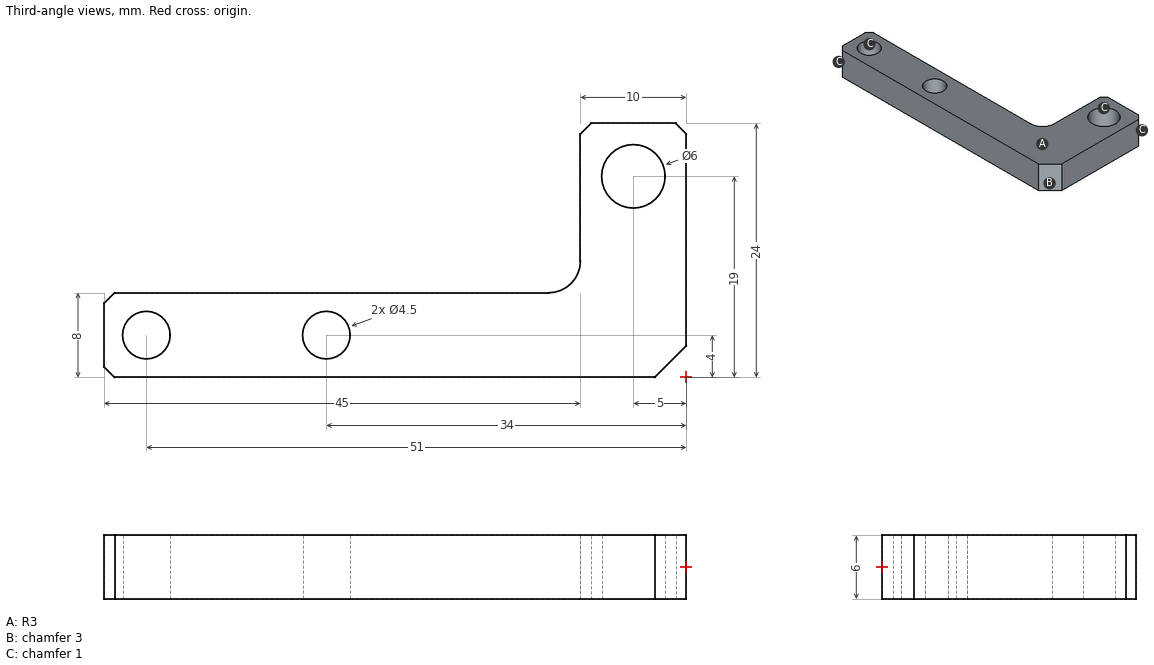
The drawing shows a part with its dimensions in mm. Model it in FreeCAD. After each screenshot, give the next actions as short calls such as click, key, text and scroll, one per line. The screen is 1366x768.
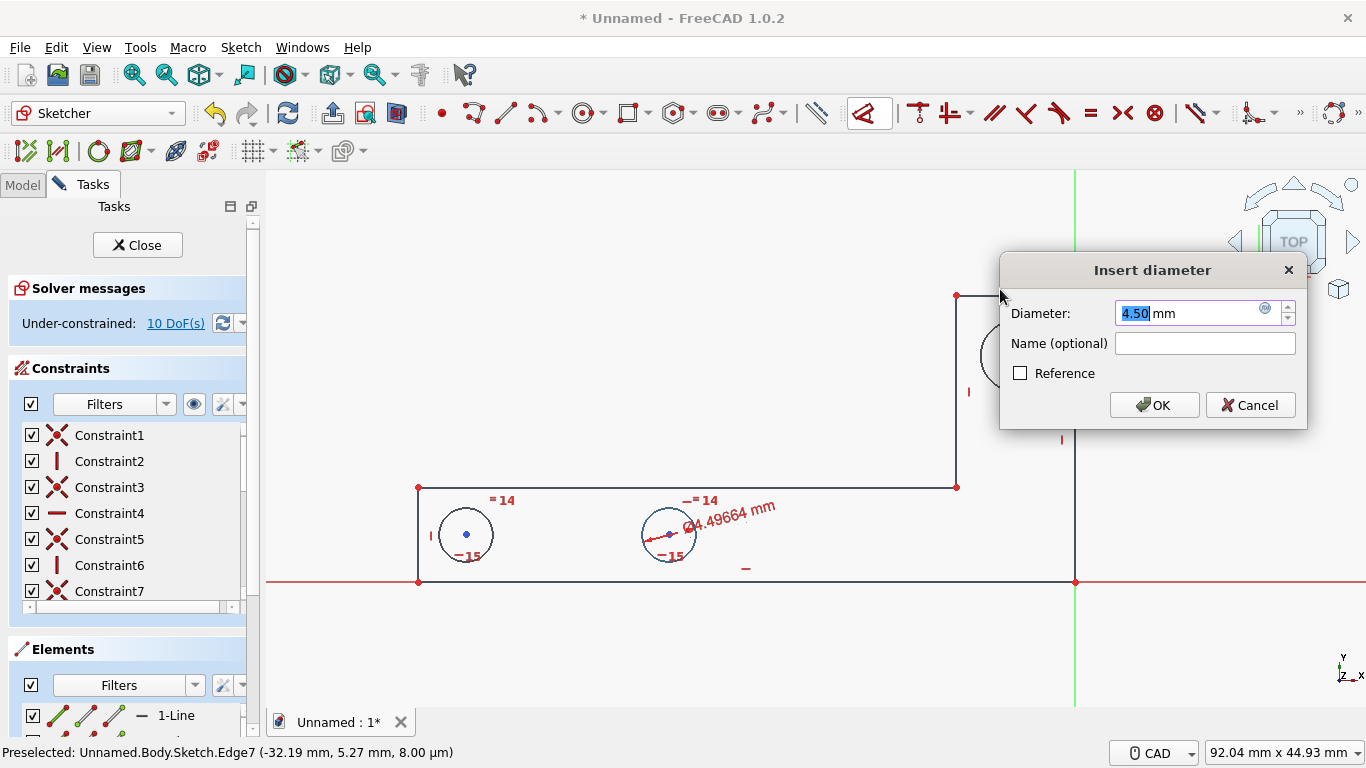
text(4.5)
key(Return)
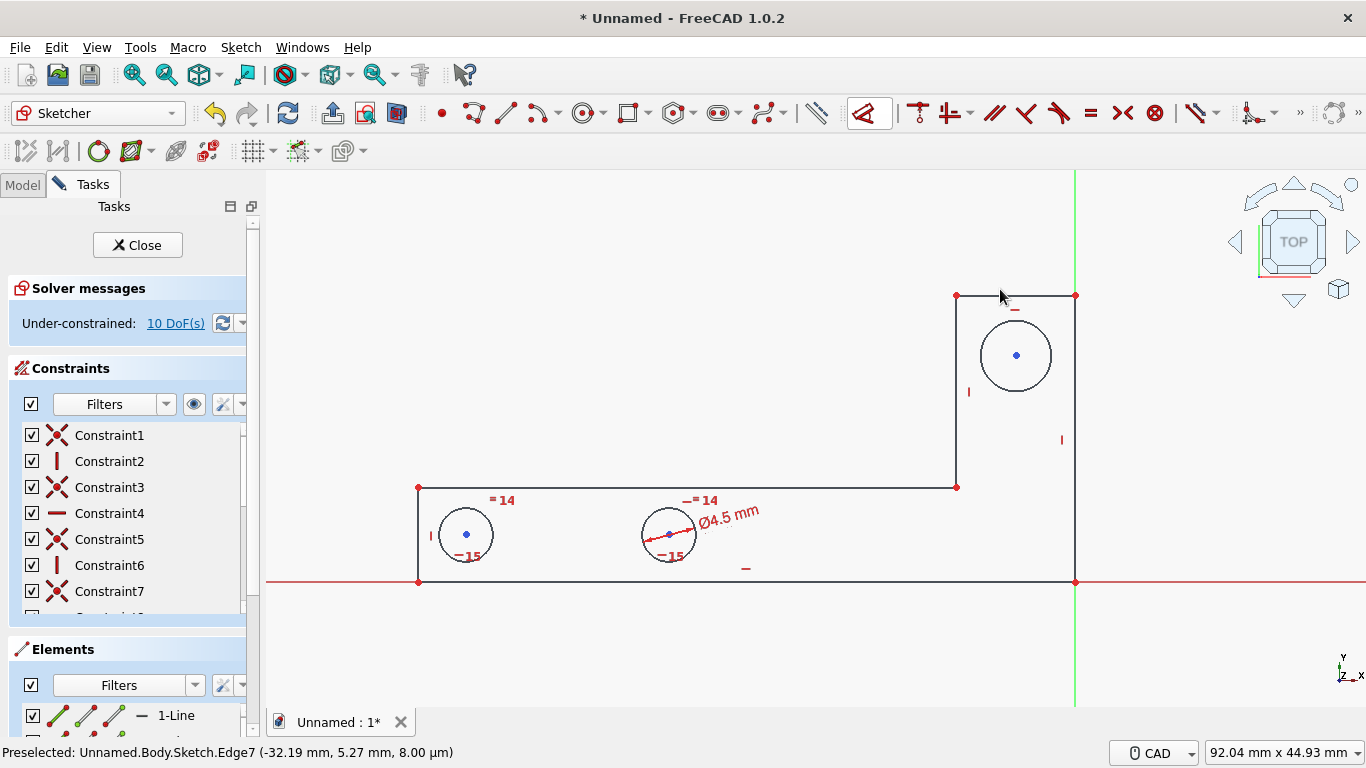
click(1041, 331)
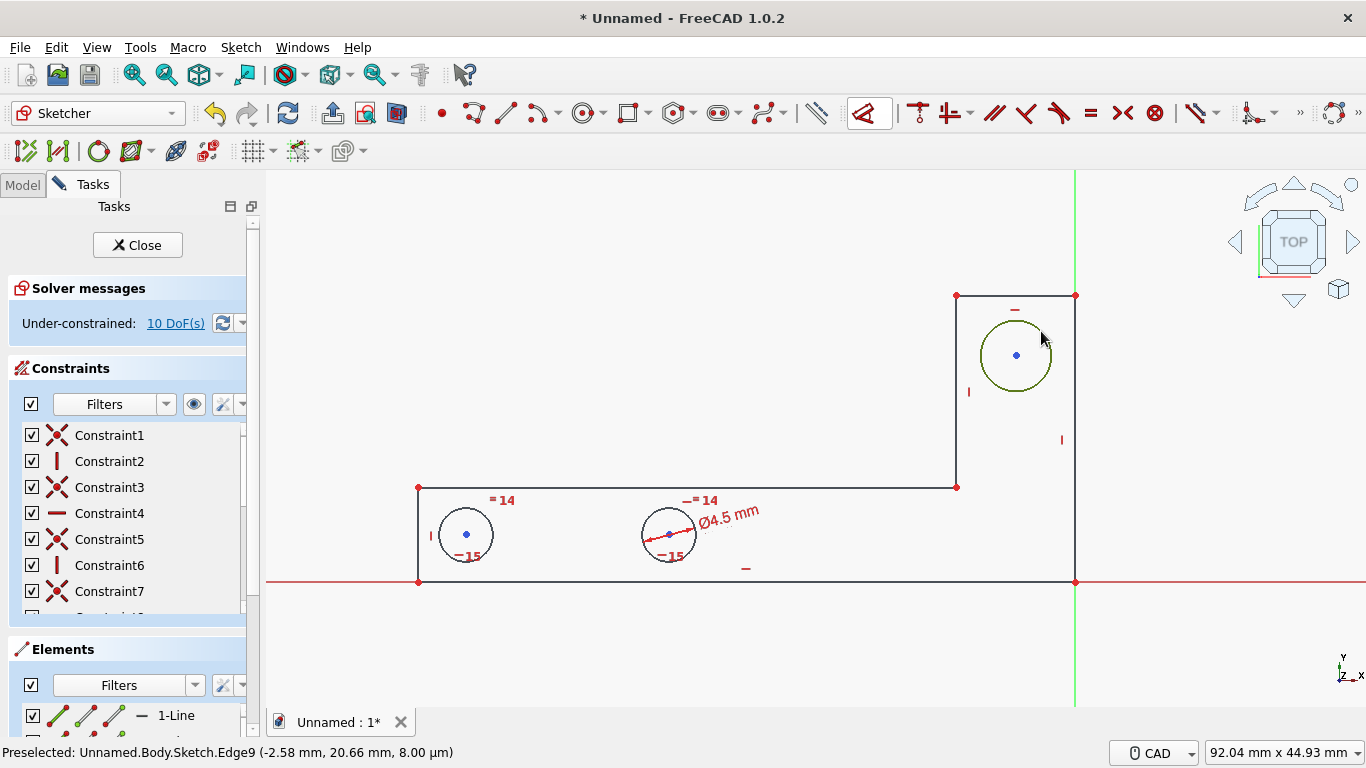
key(k)
key(o)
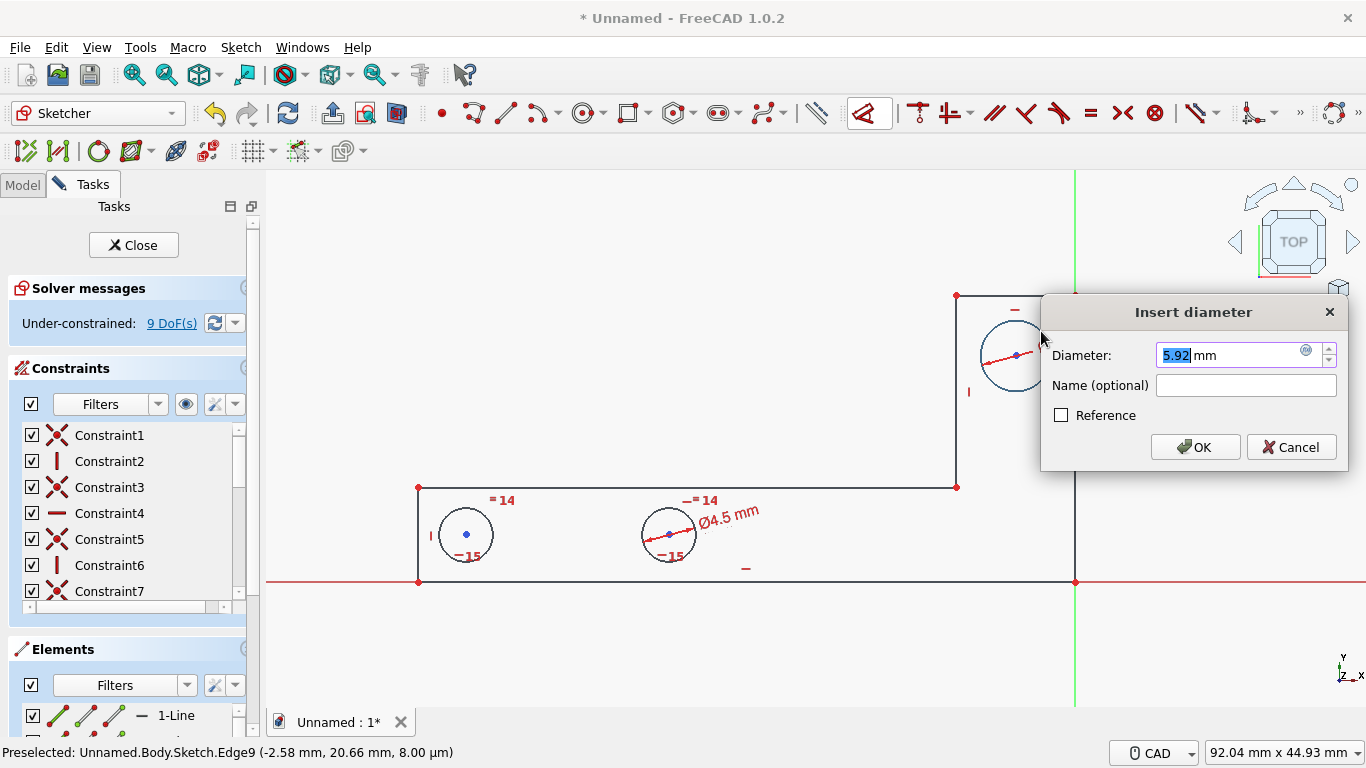
text(6)
key(Return)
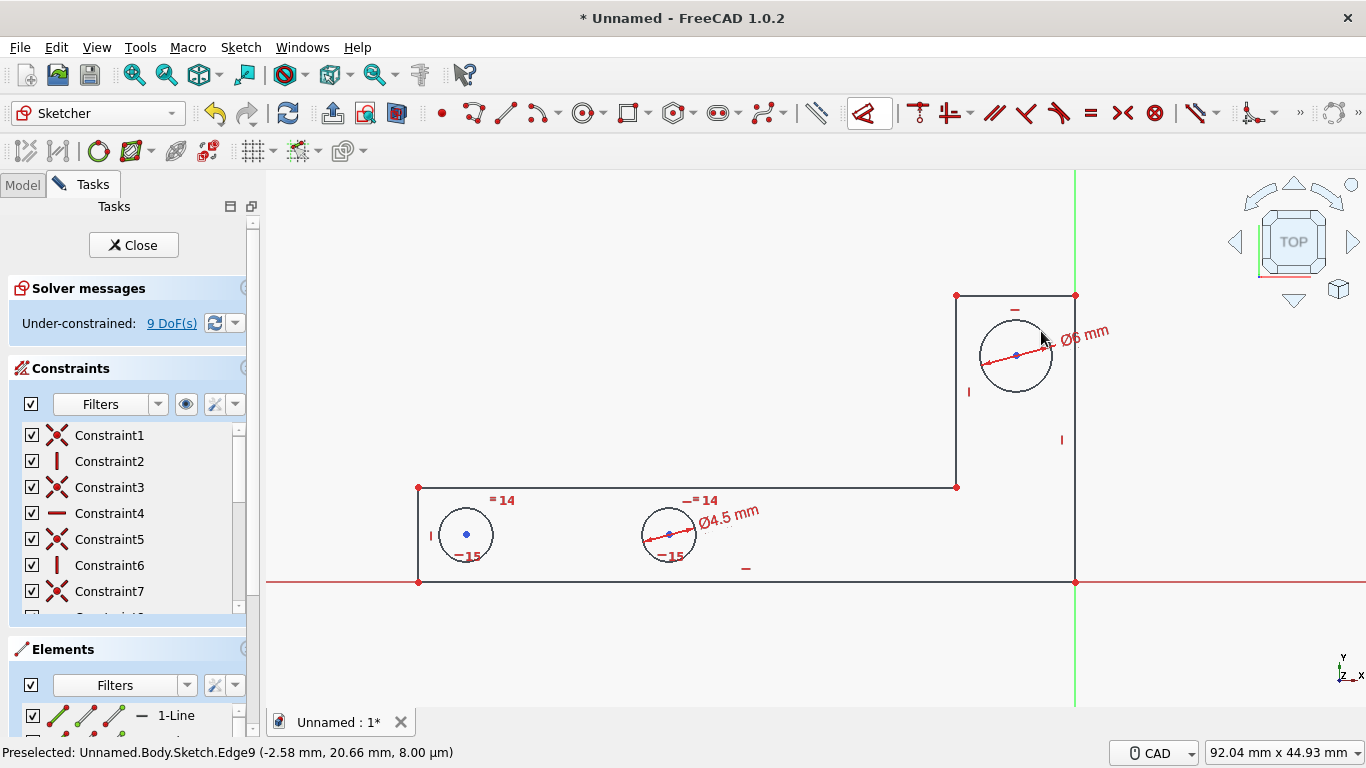
click(418, 516)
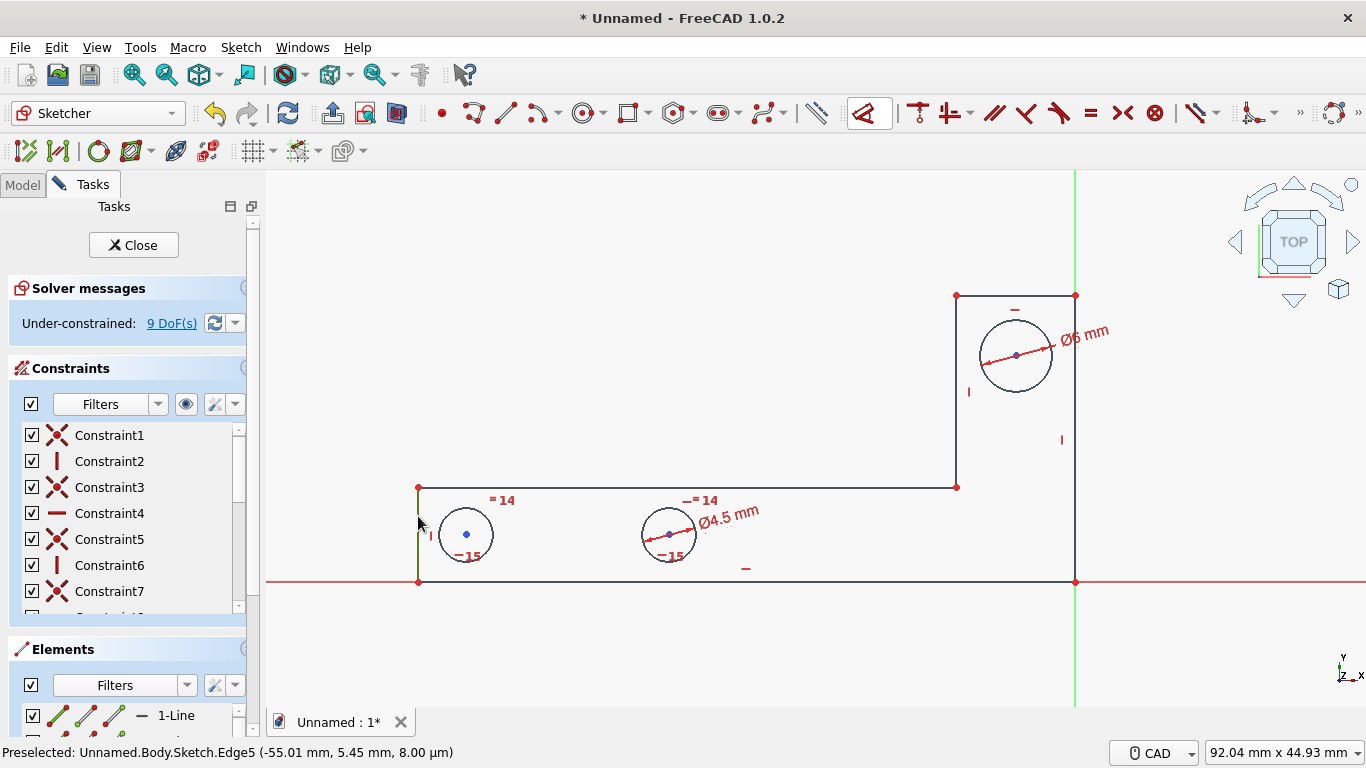
key(i)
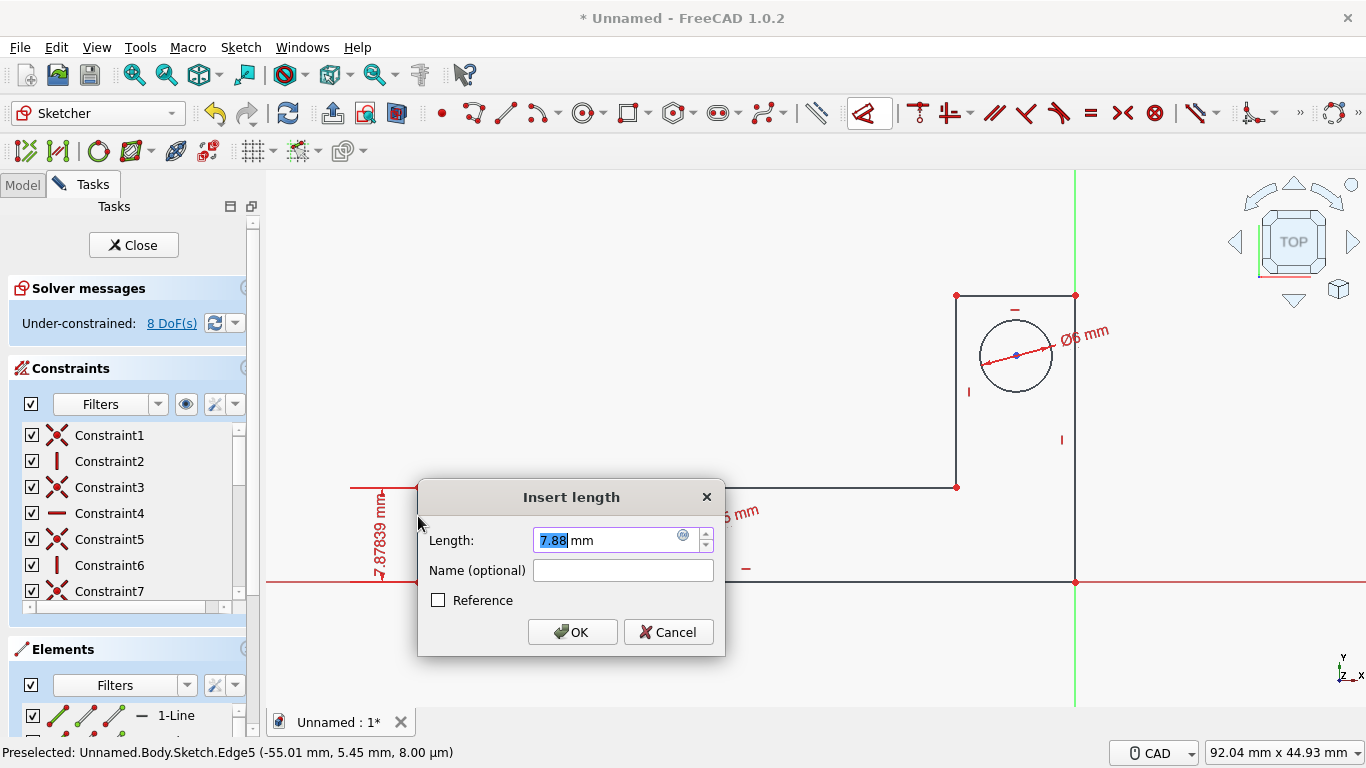
text(8)
key(Return)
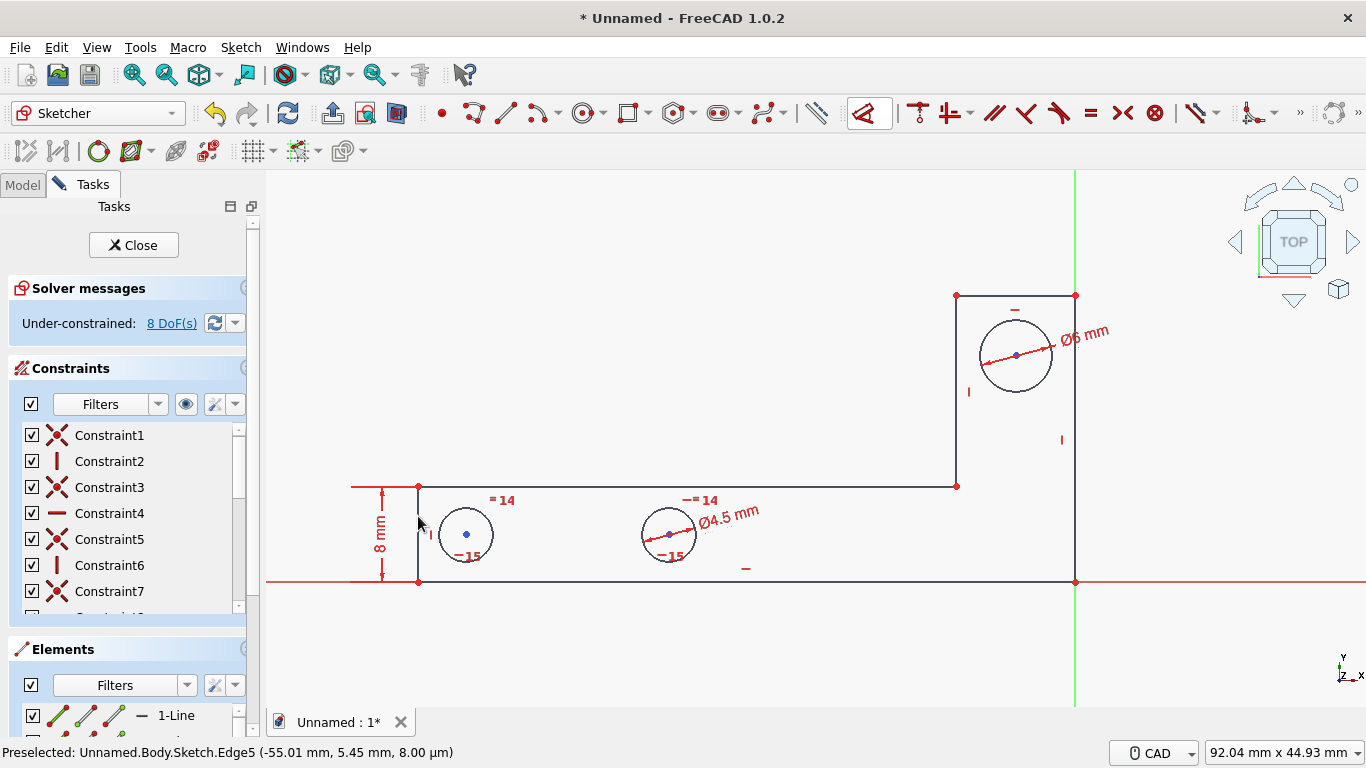
click(669, 535)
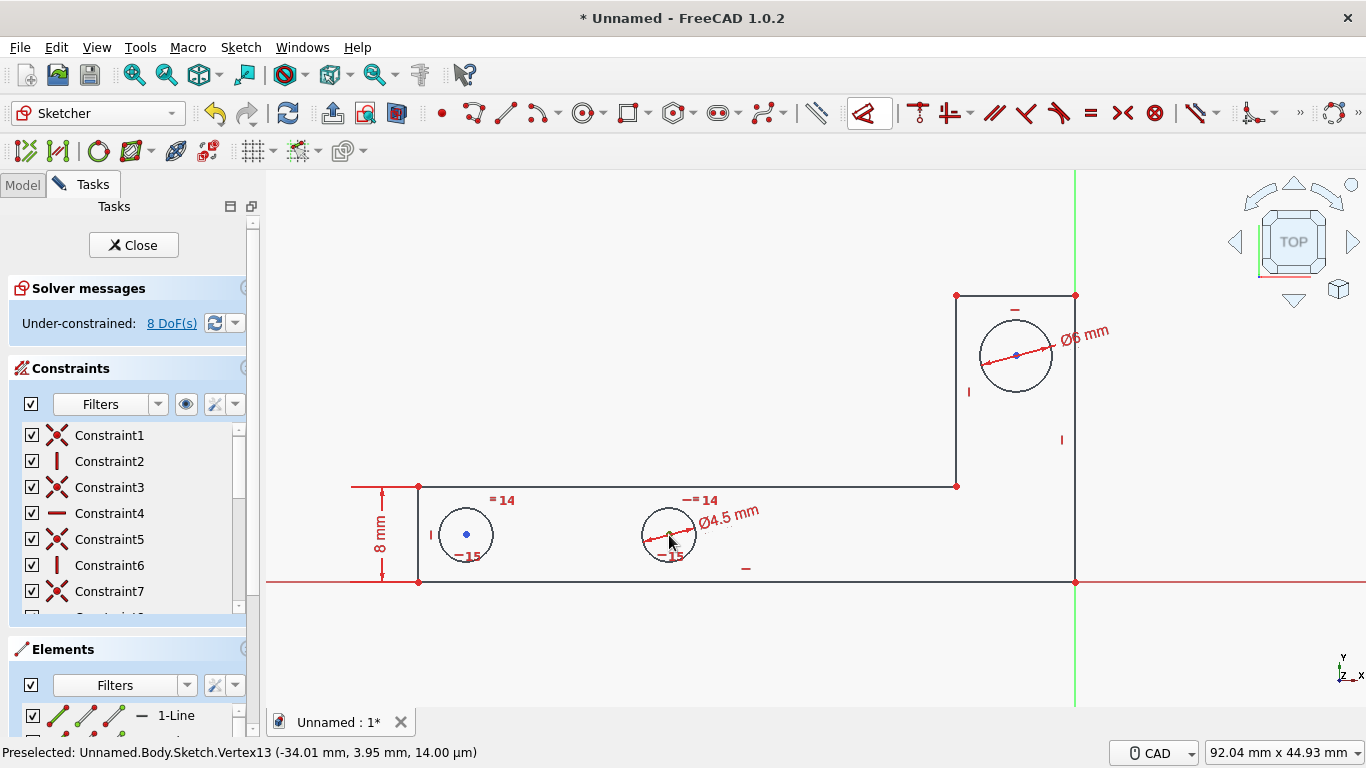
key(i)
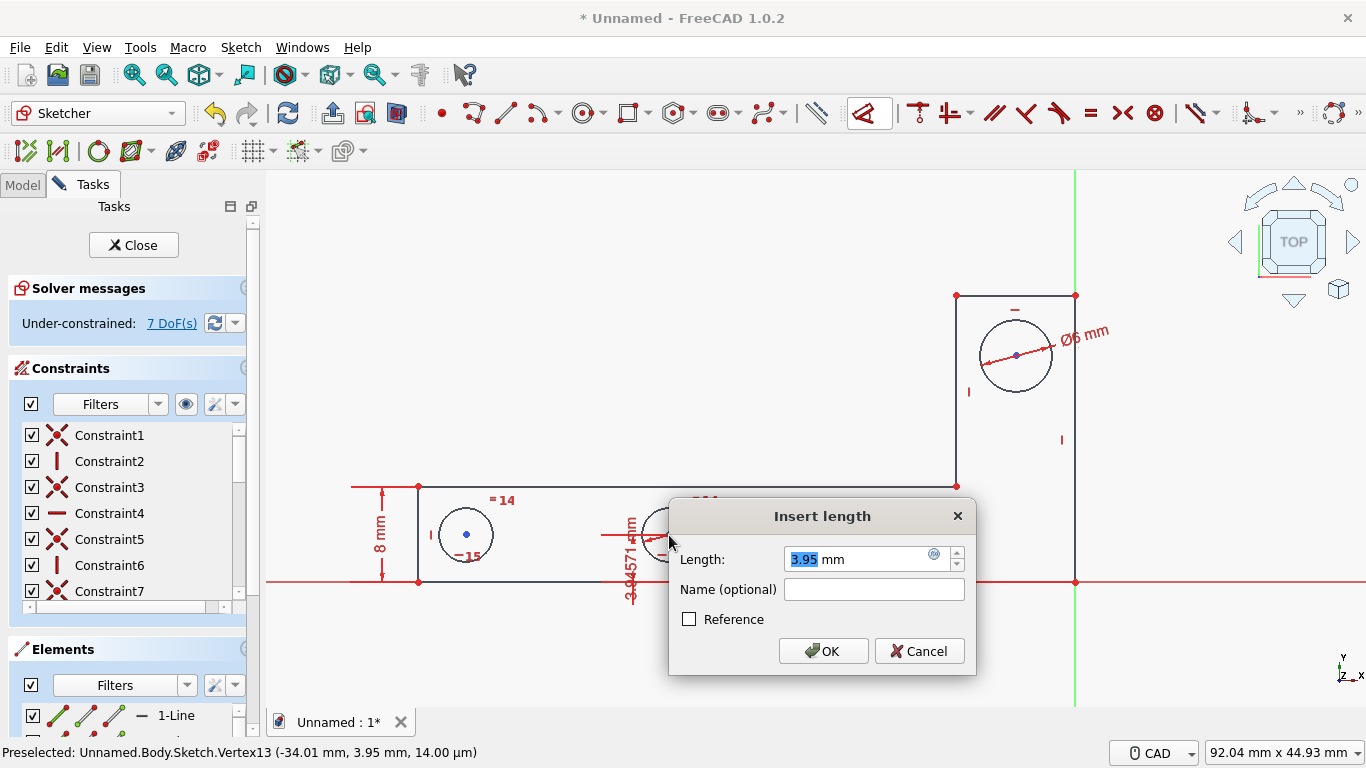
text(4)
key(Return)